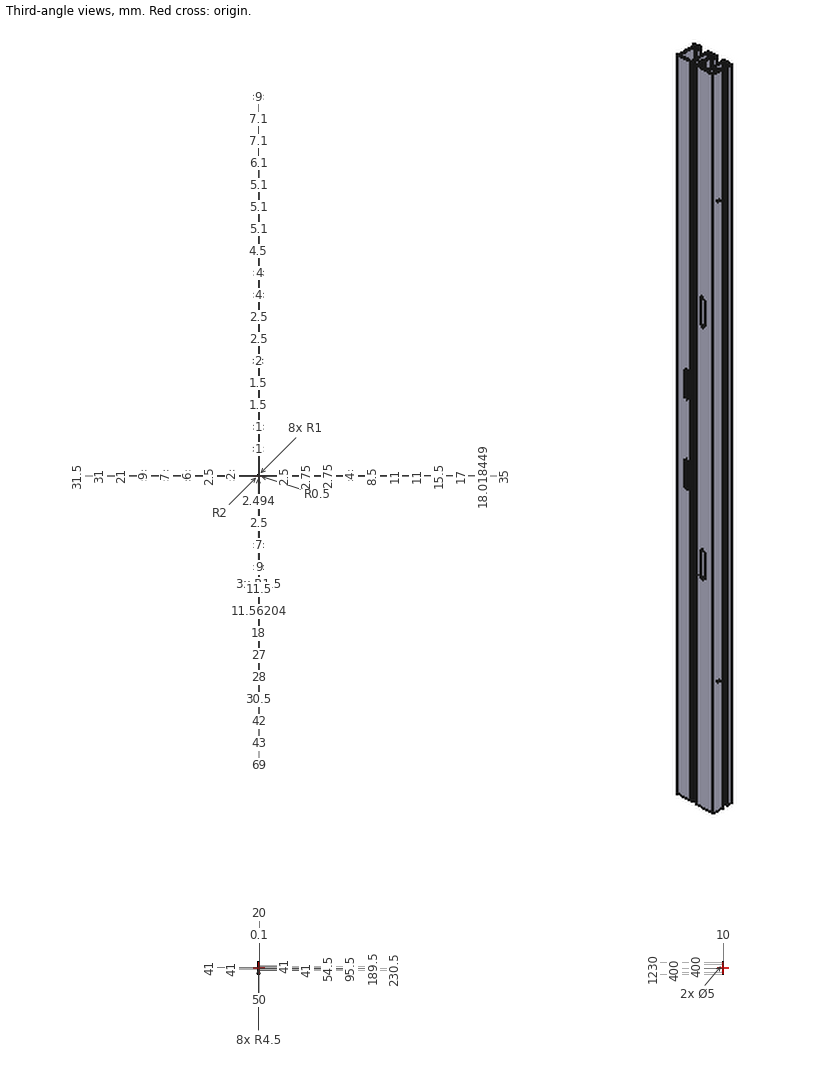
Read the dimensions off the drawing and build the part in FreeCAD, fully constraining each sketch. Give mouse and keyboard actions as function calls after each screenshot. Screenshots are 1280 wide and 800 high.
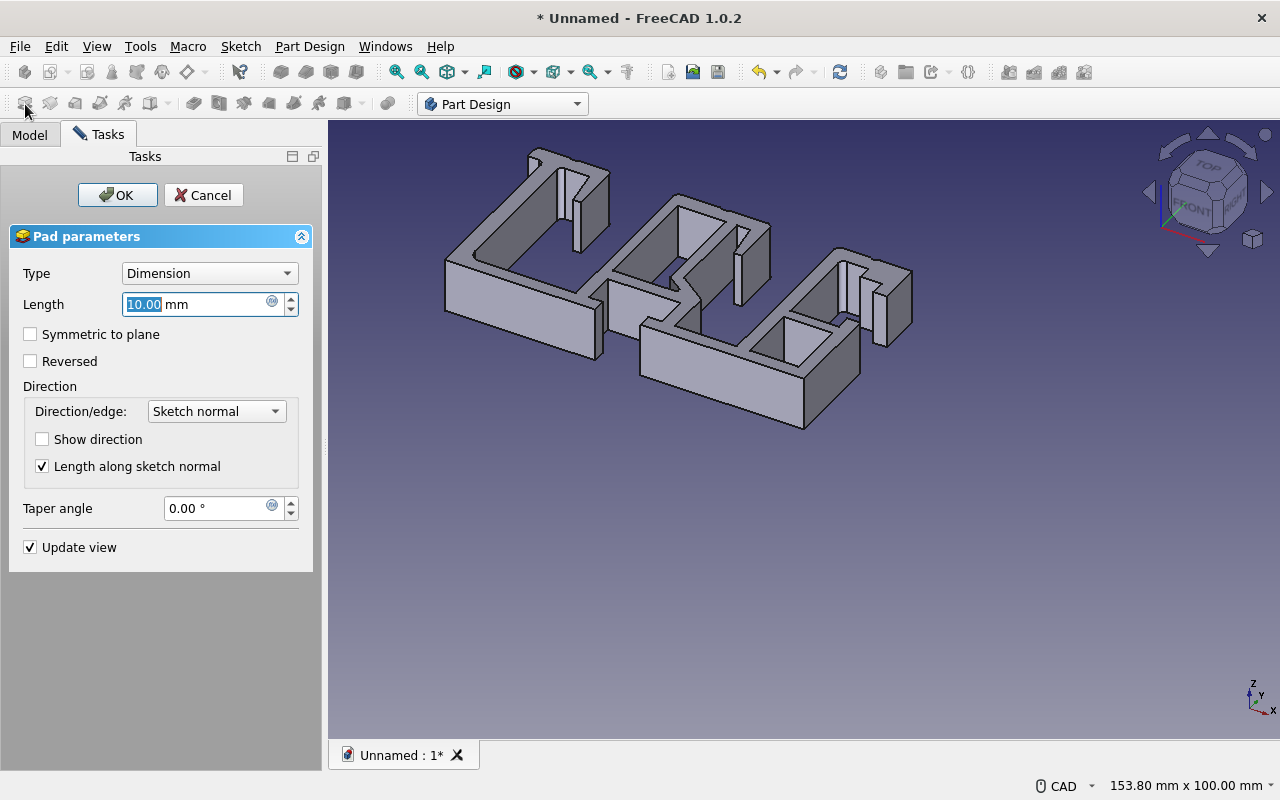
text(1230)
key(Tab)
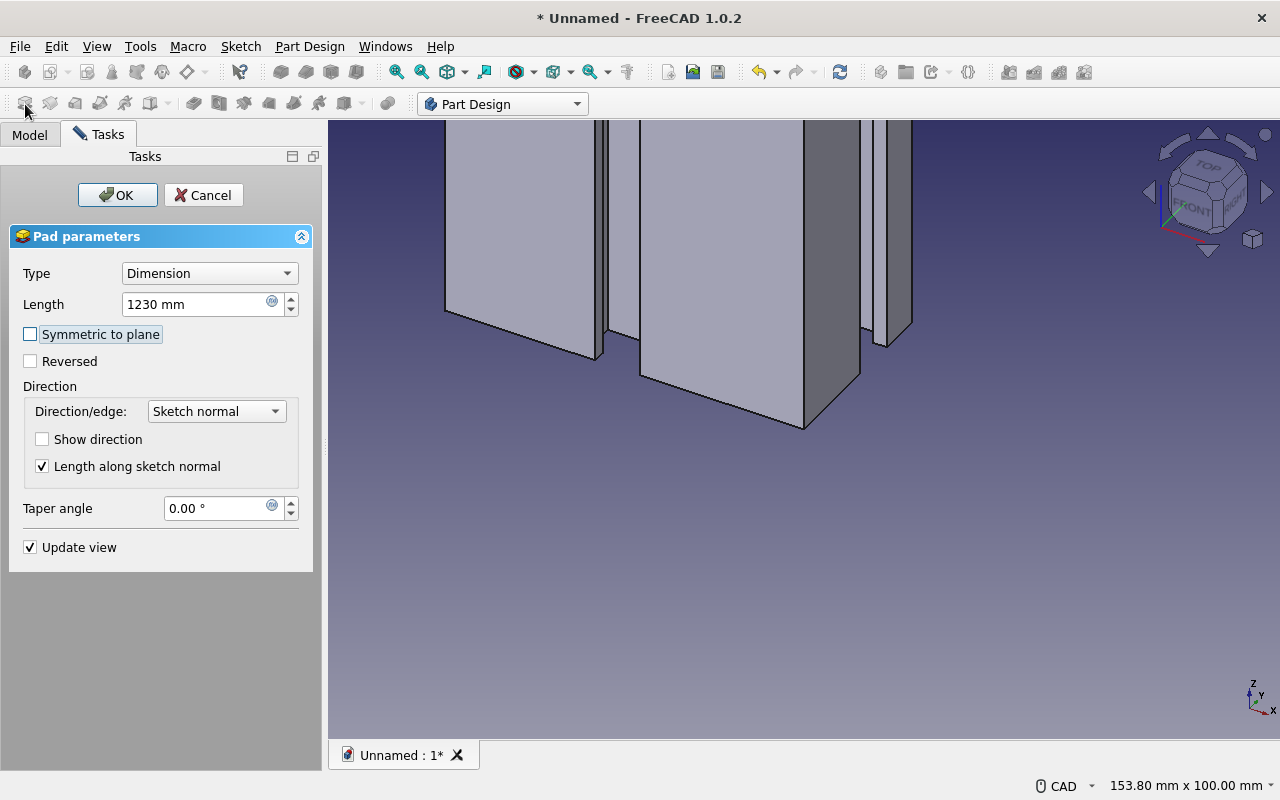
click(31, 334)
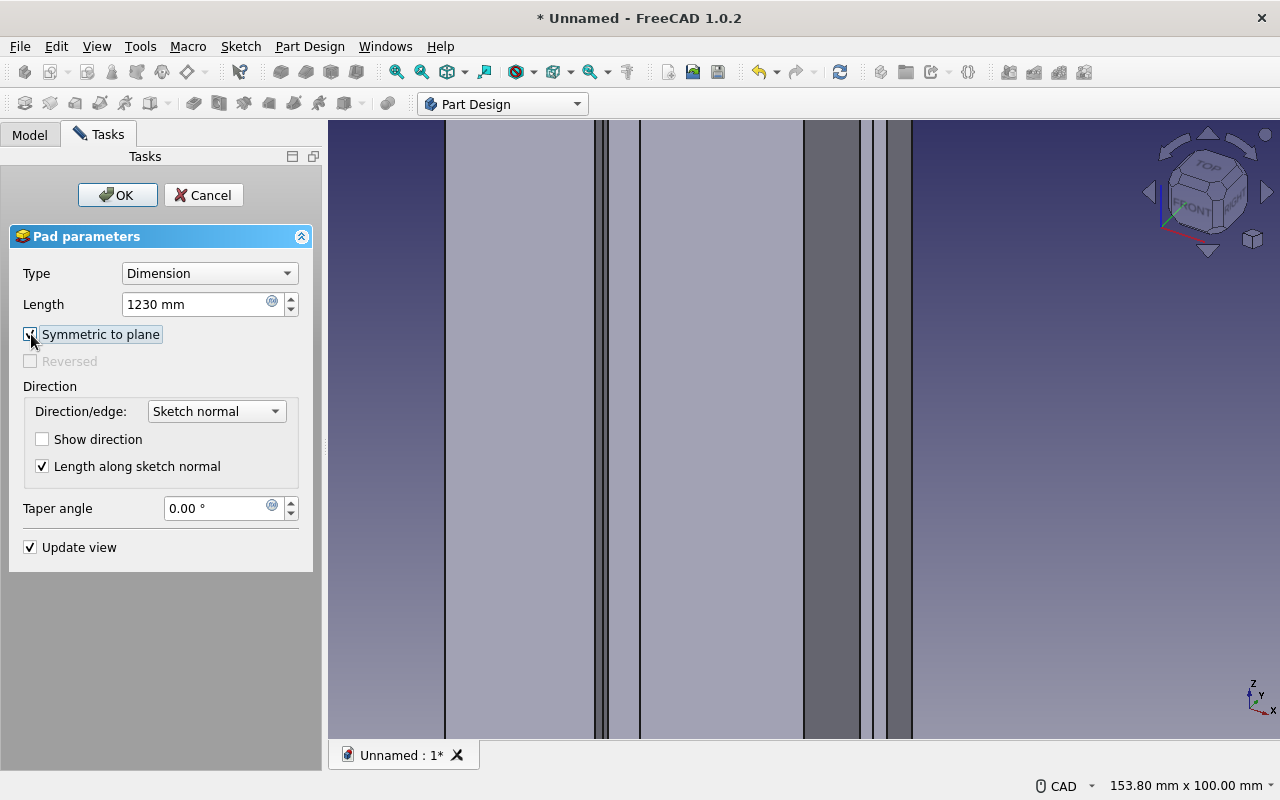
click(118, 195)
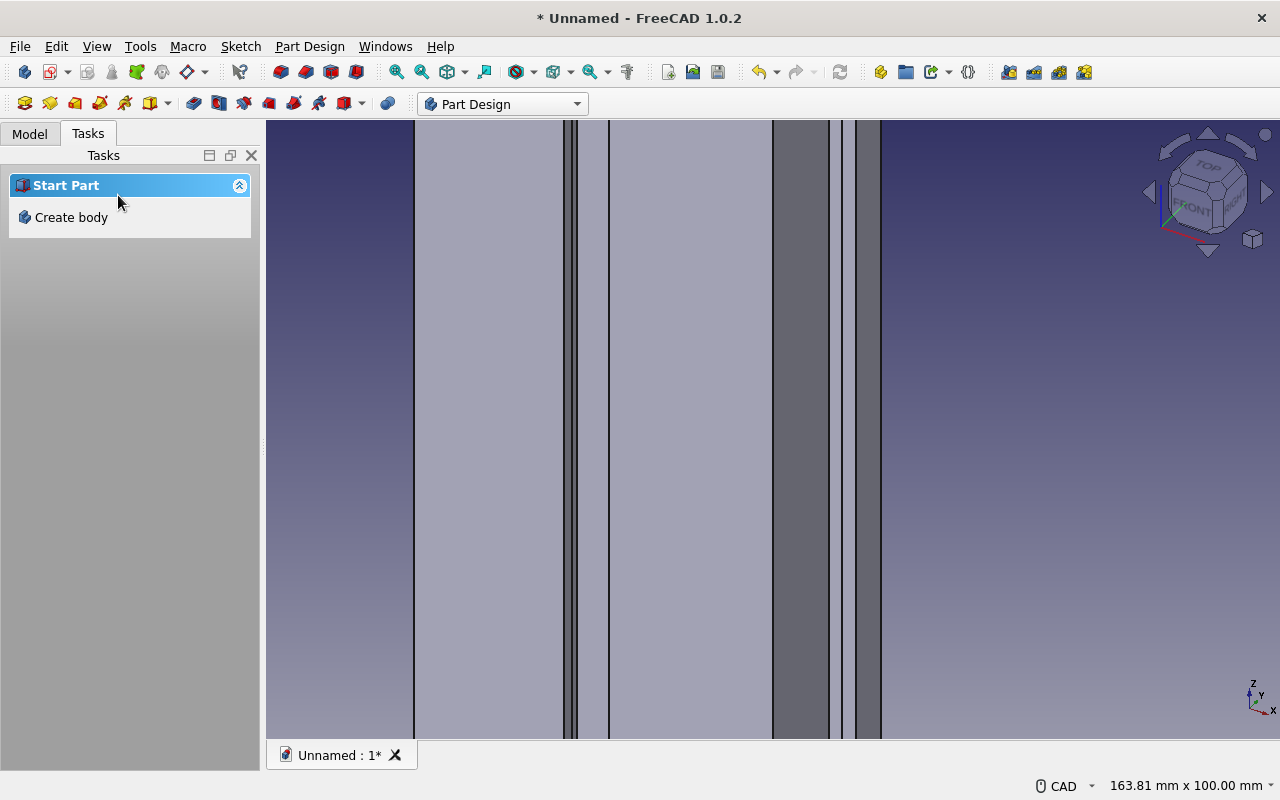
click(397, 72)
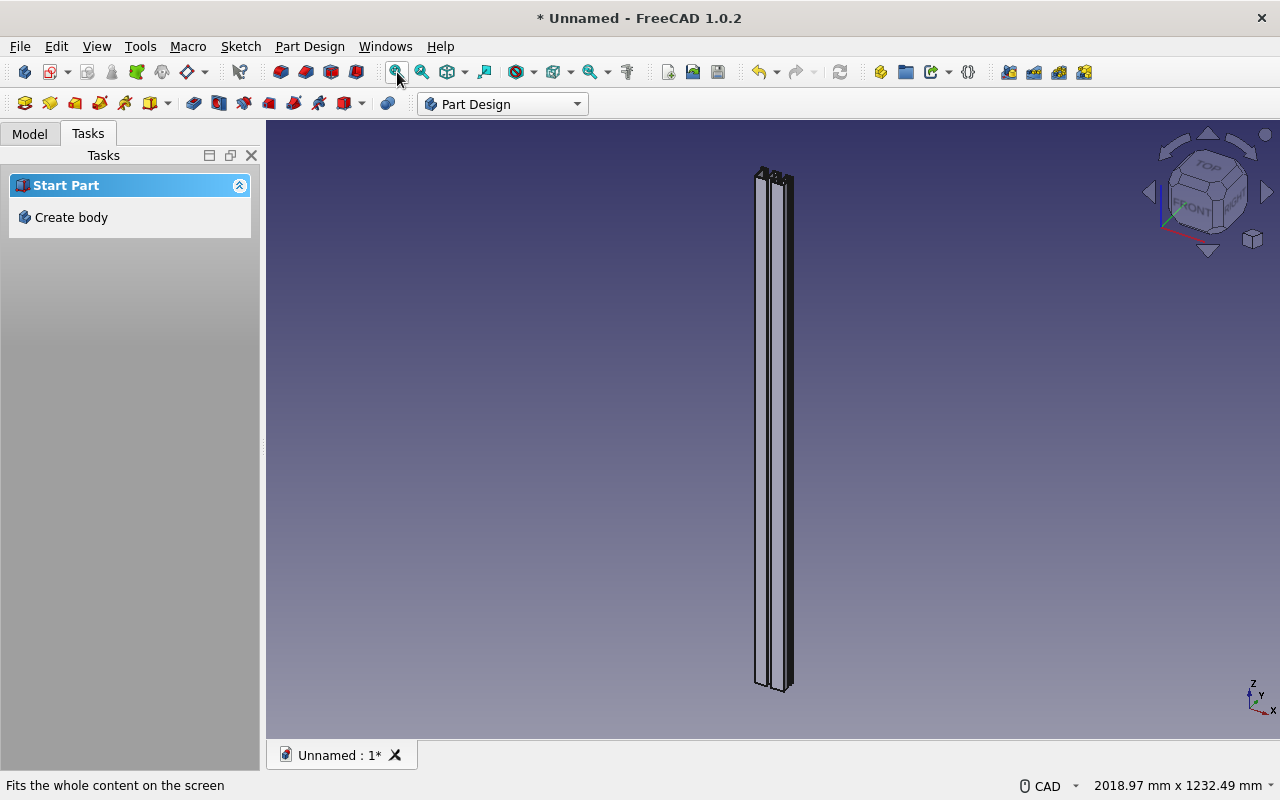
key(4)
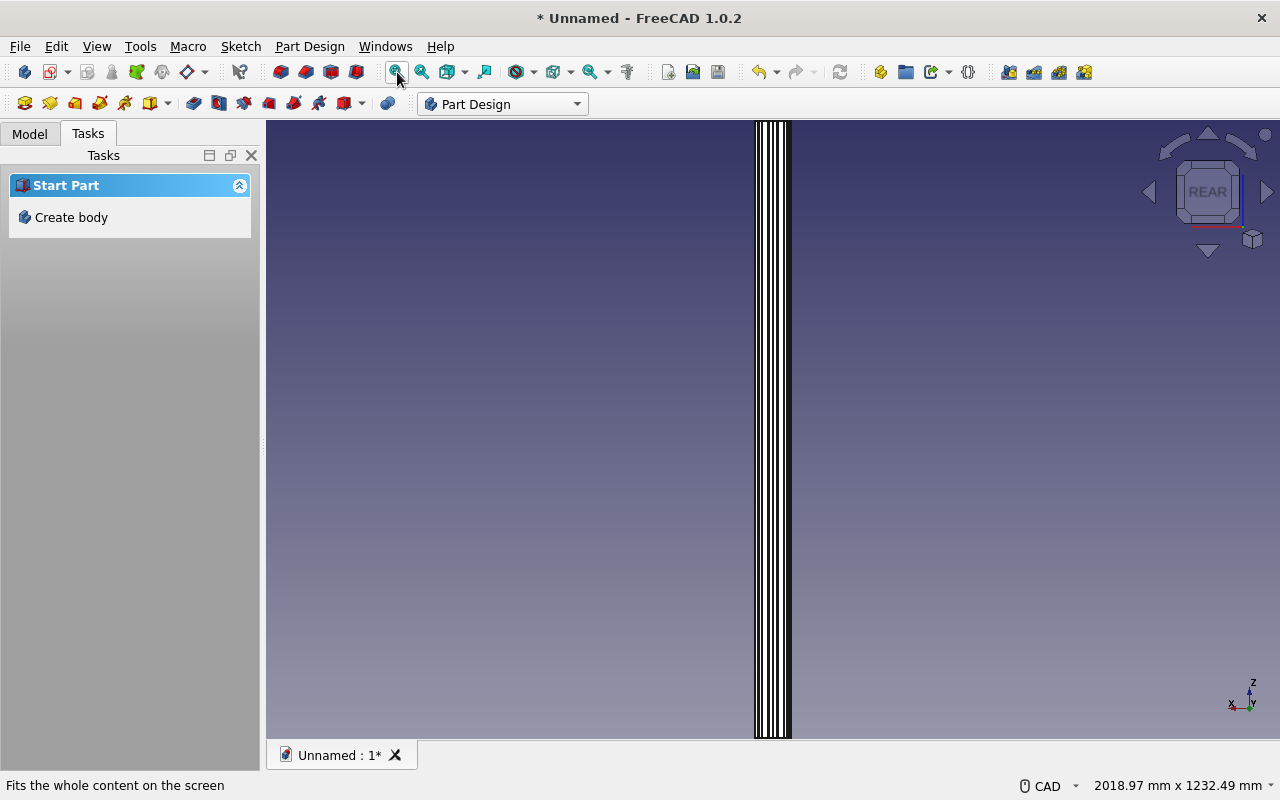
scroll(782, 164, up, 5)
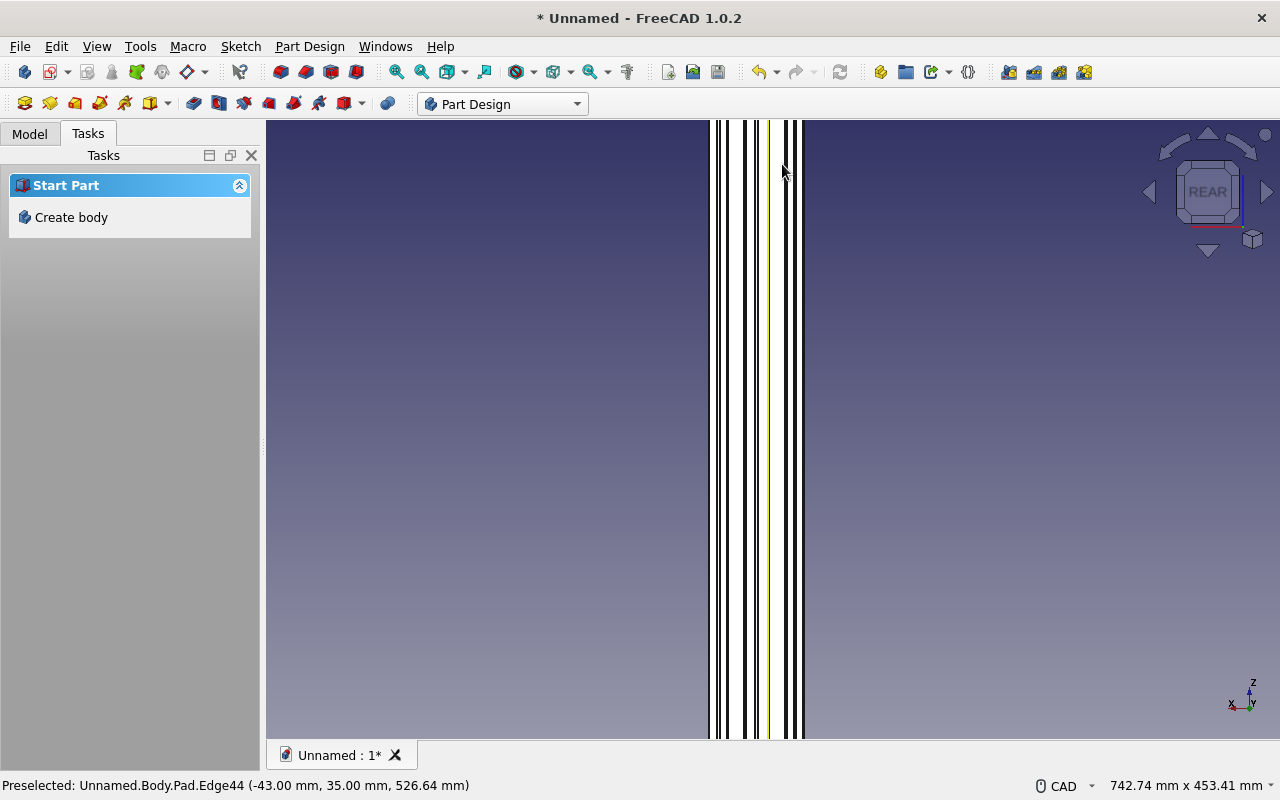
click(397, 72)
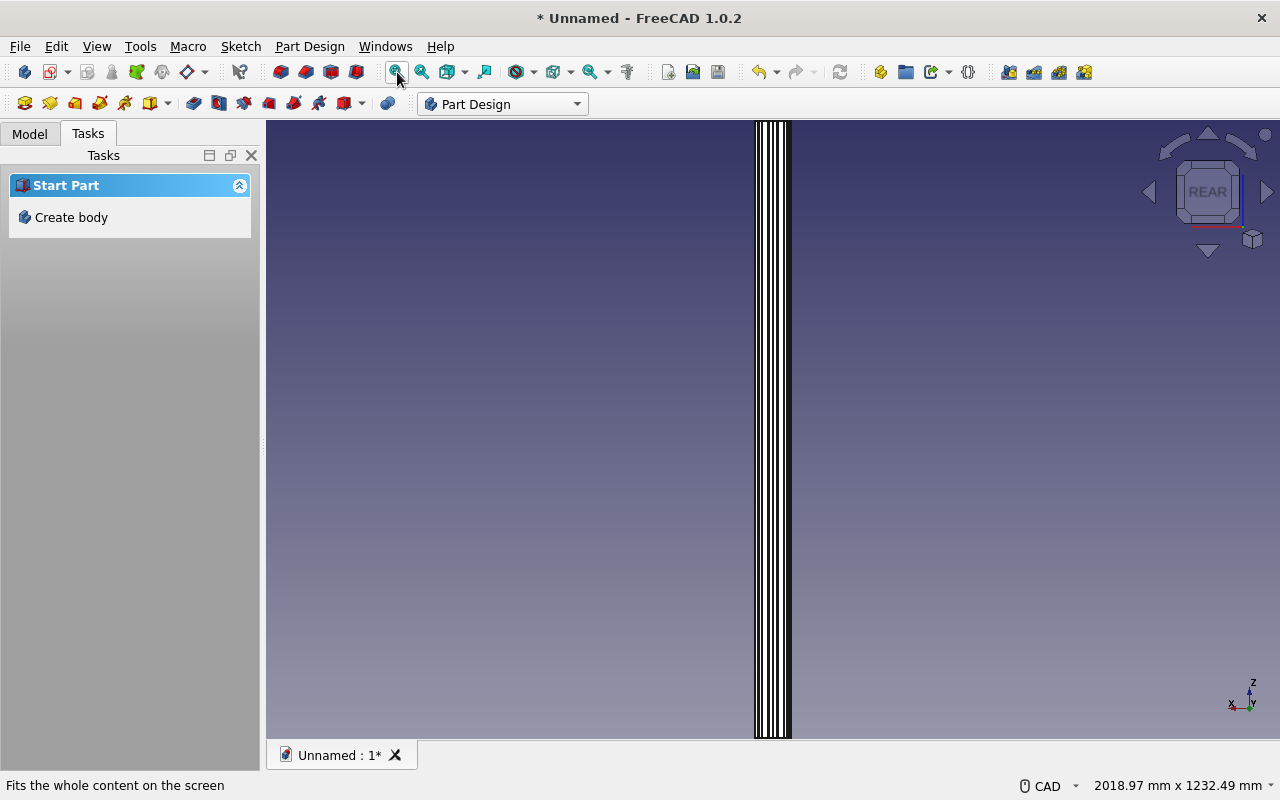
key(2)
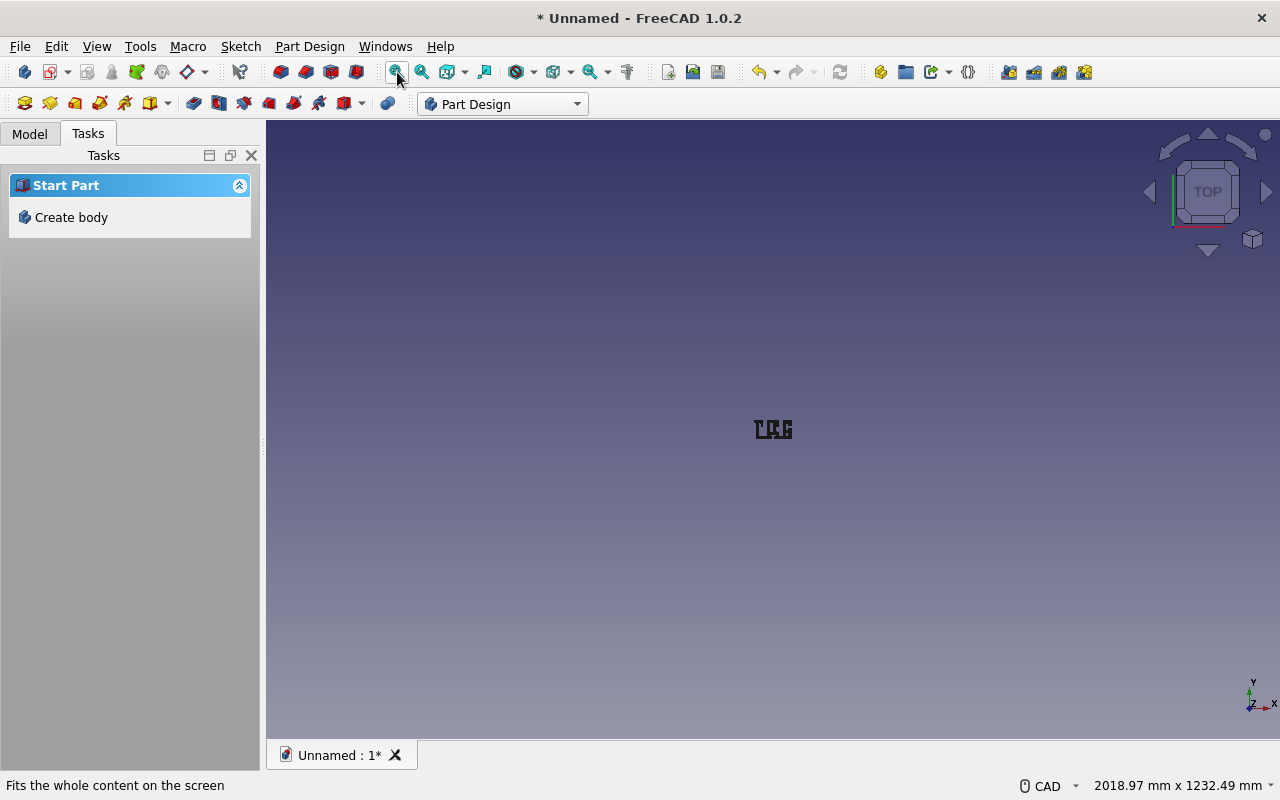
click(397, 72)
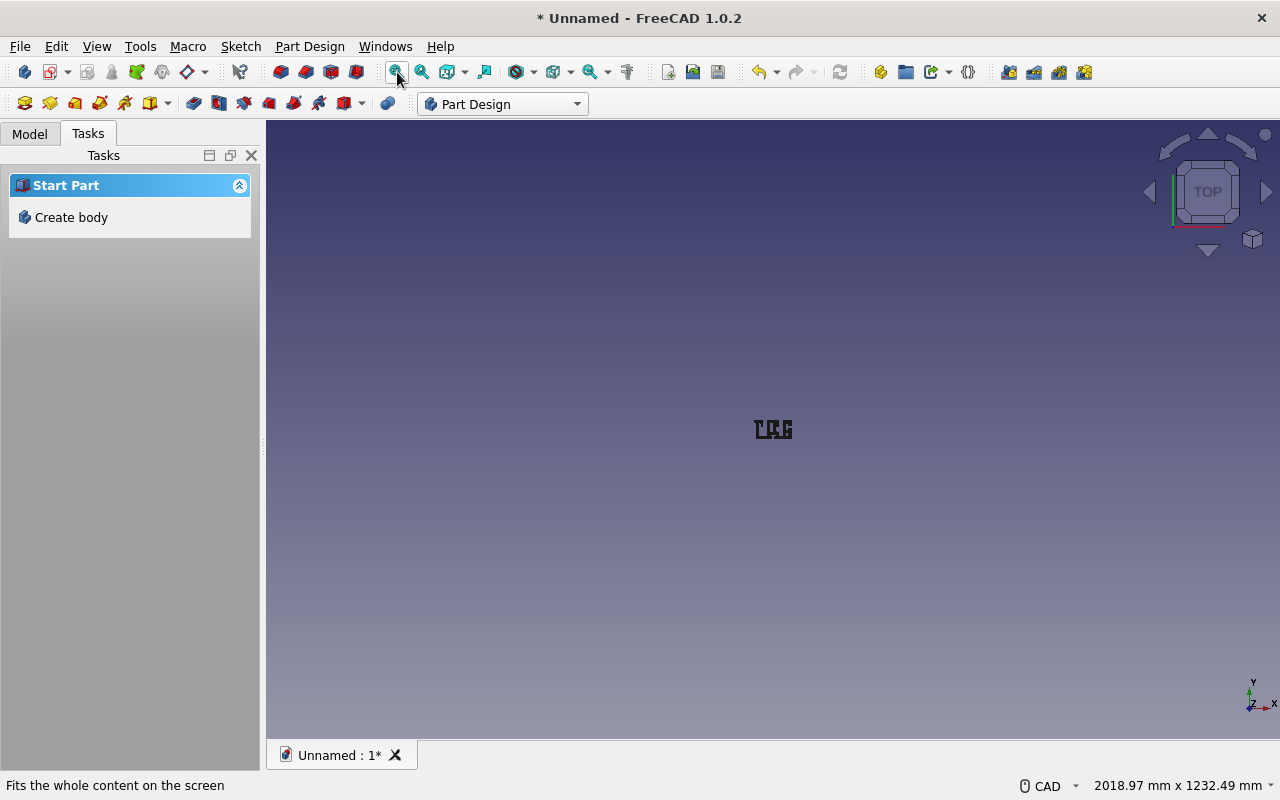
key(3)